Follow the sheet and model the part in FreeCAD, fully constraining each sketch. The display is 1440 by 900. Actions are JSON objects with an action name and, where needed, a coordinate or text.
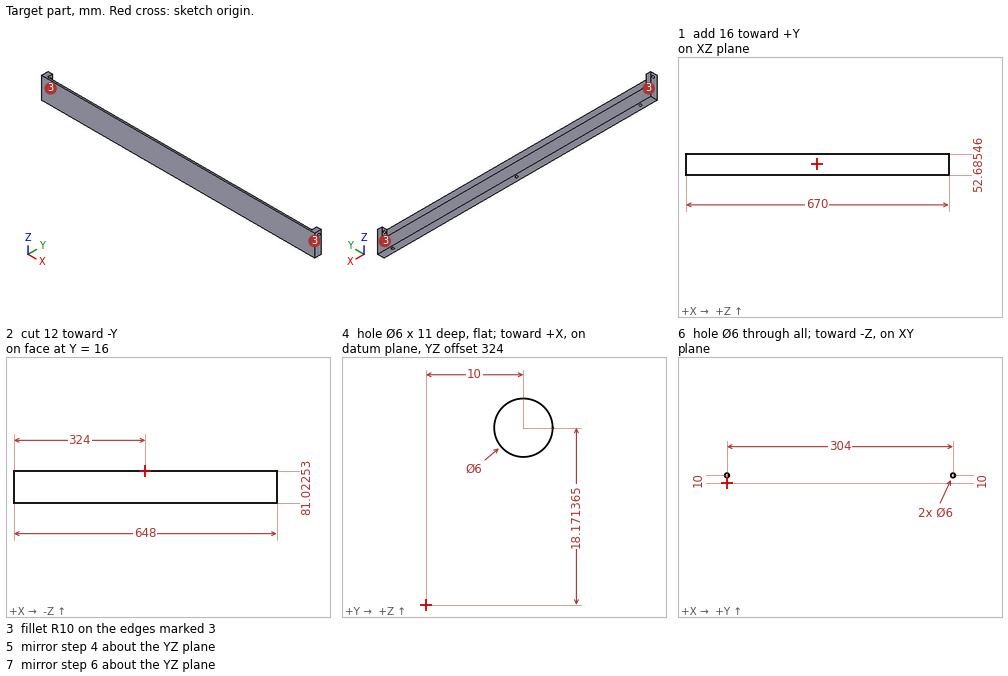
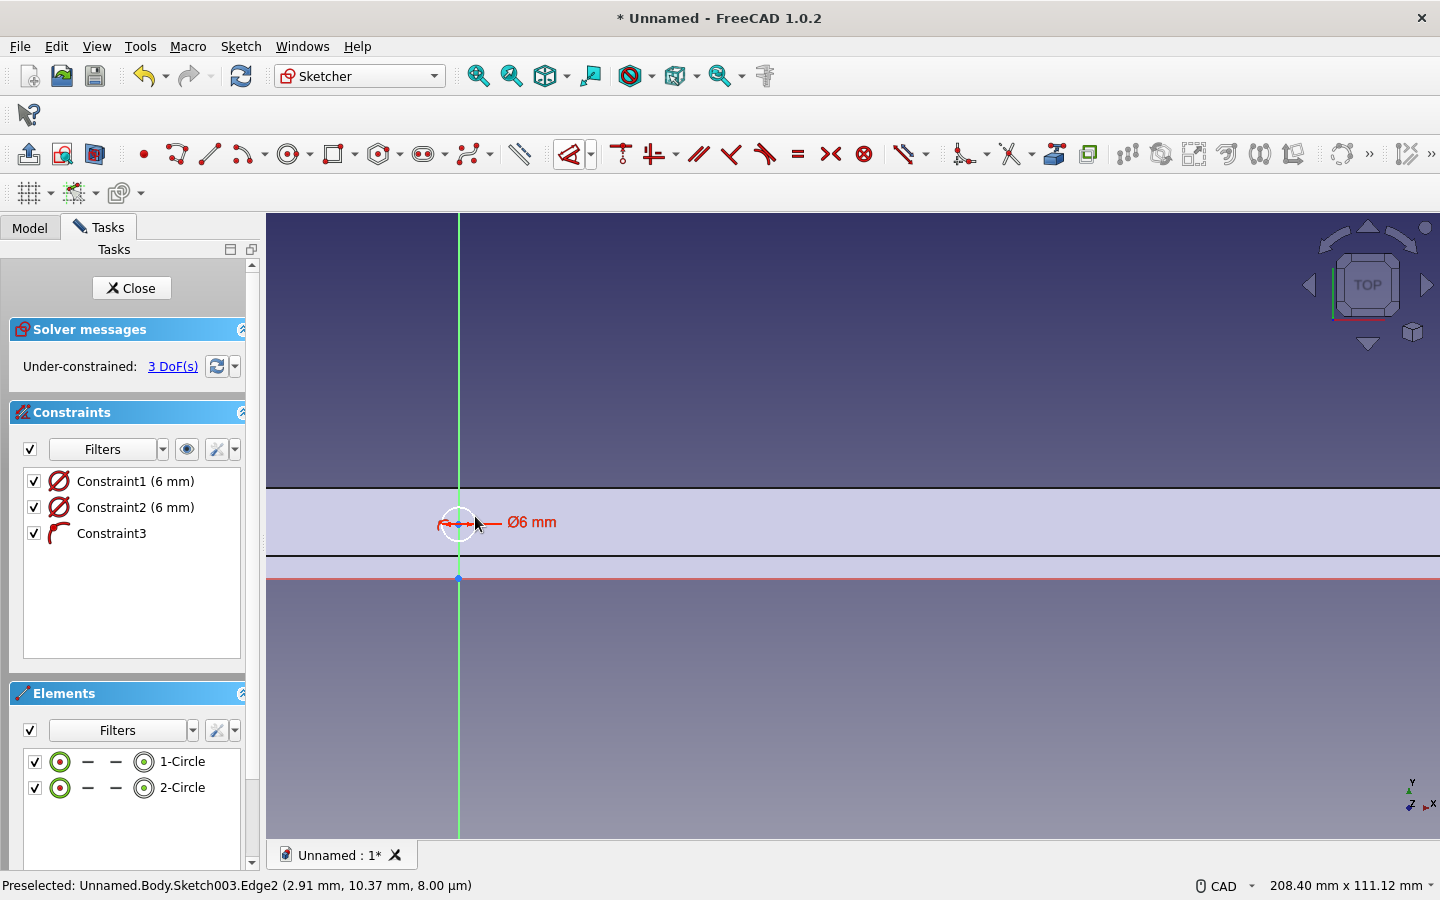
{"action": "scroll", "coordinate": [476, 517], "scroll_direction": "down", "scroll_amount": 5}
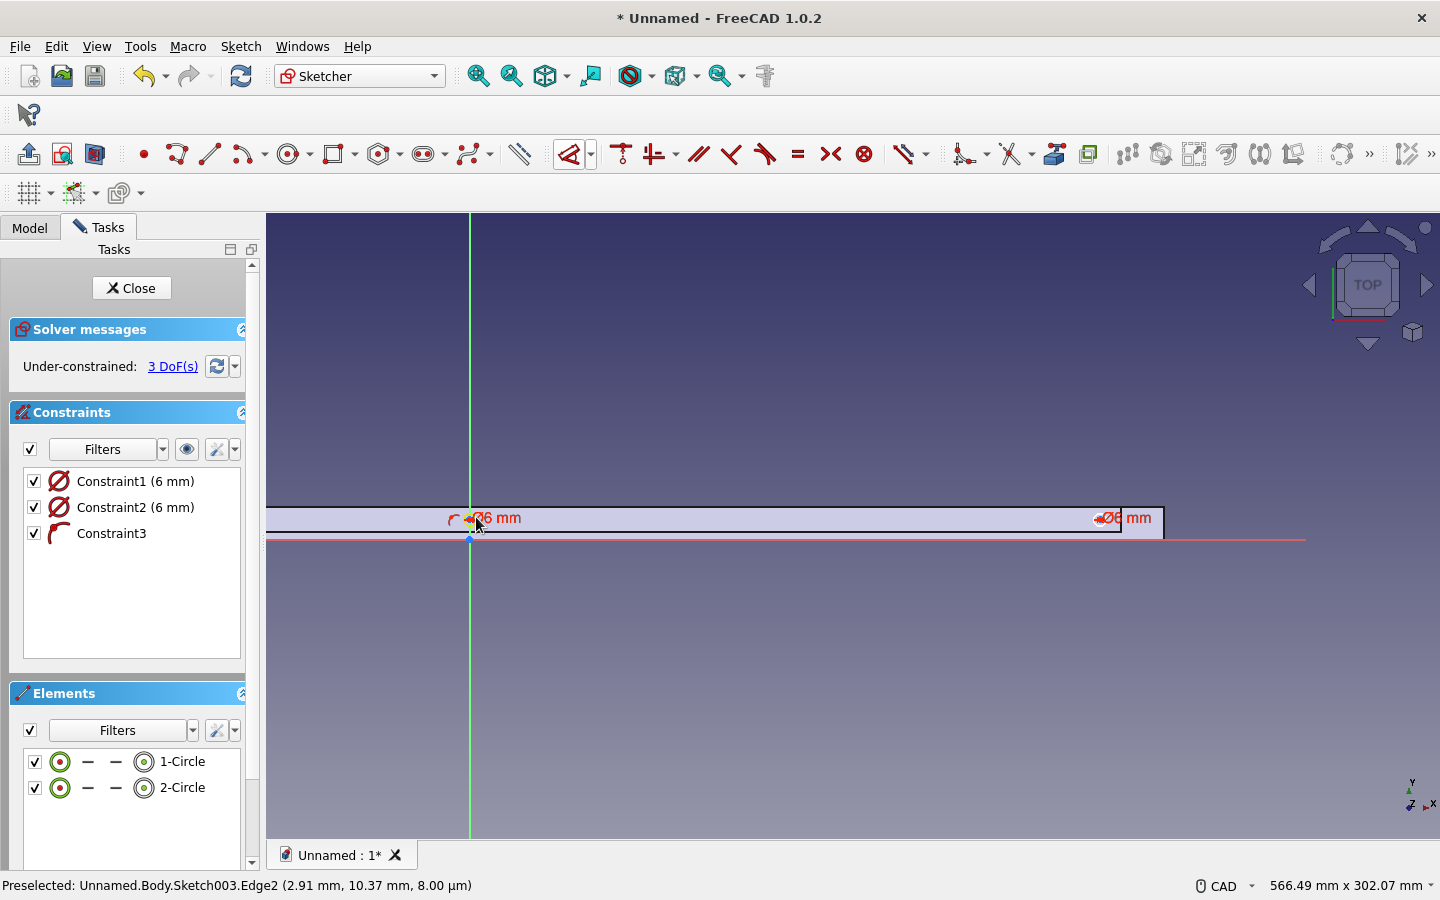
{"action": "scroll", "coordinate": [1100, 520], "scroll_direction": "up", "scroll_amount": 4}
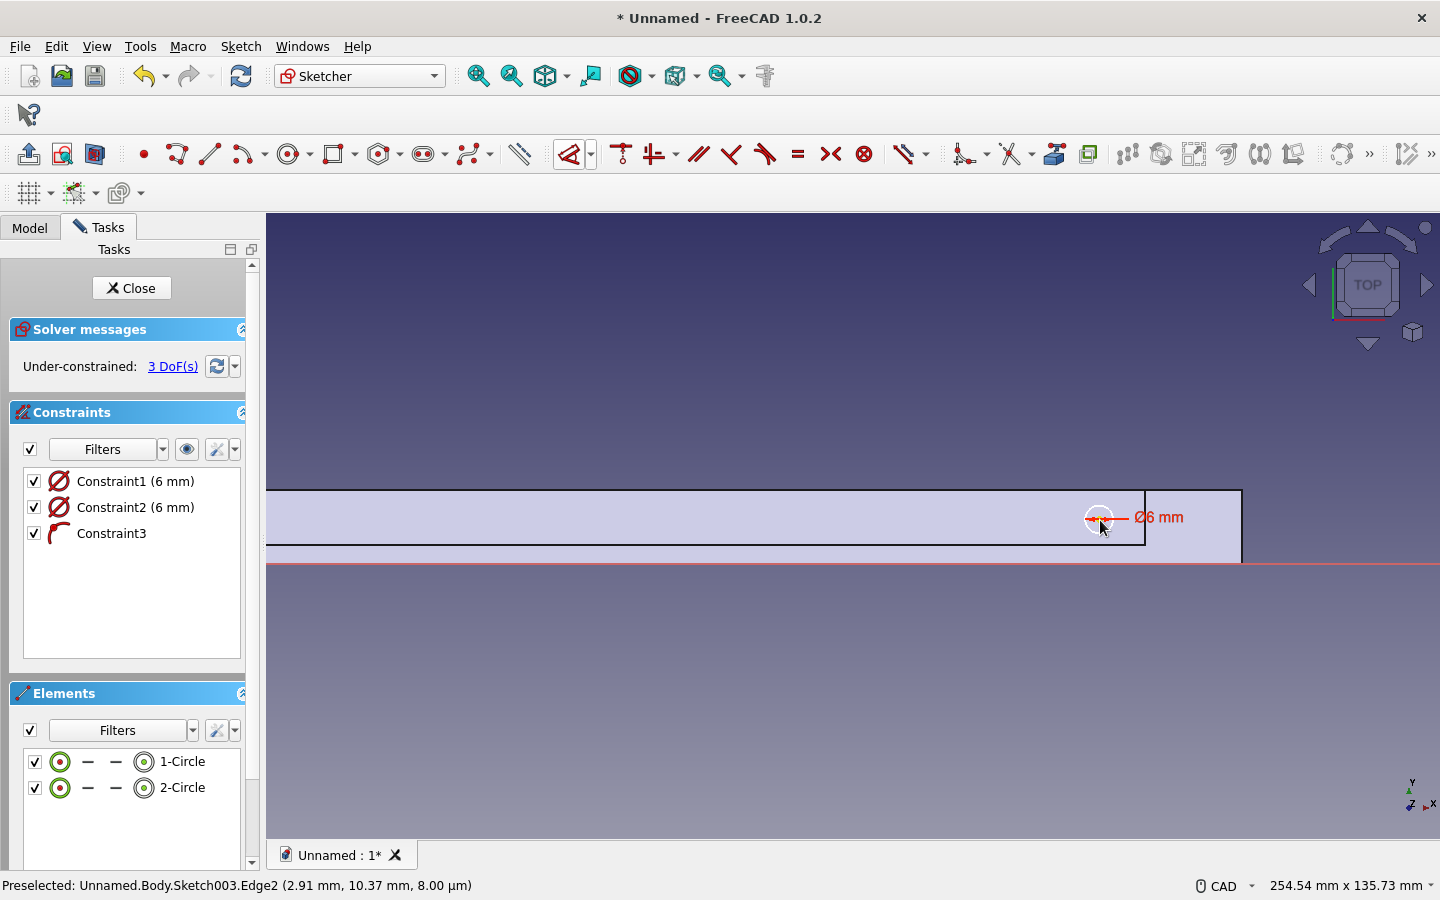
{"action": "left_click", "coordinate": [1099, 519]}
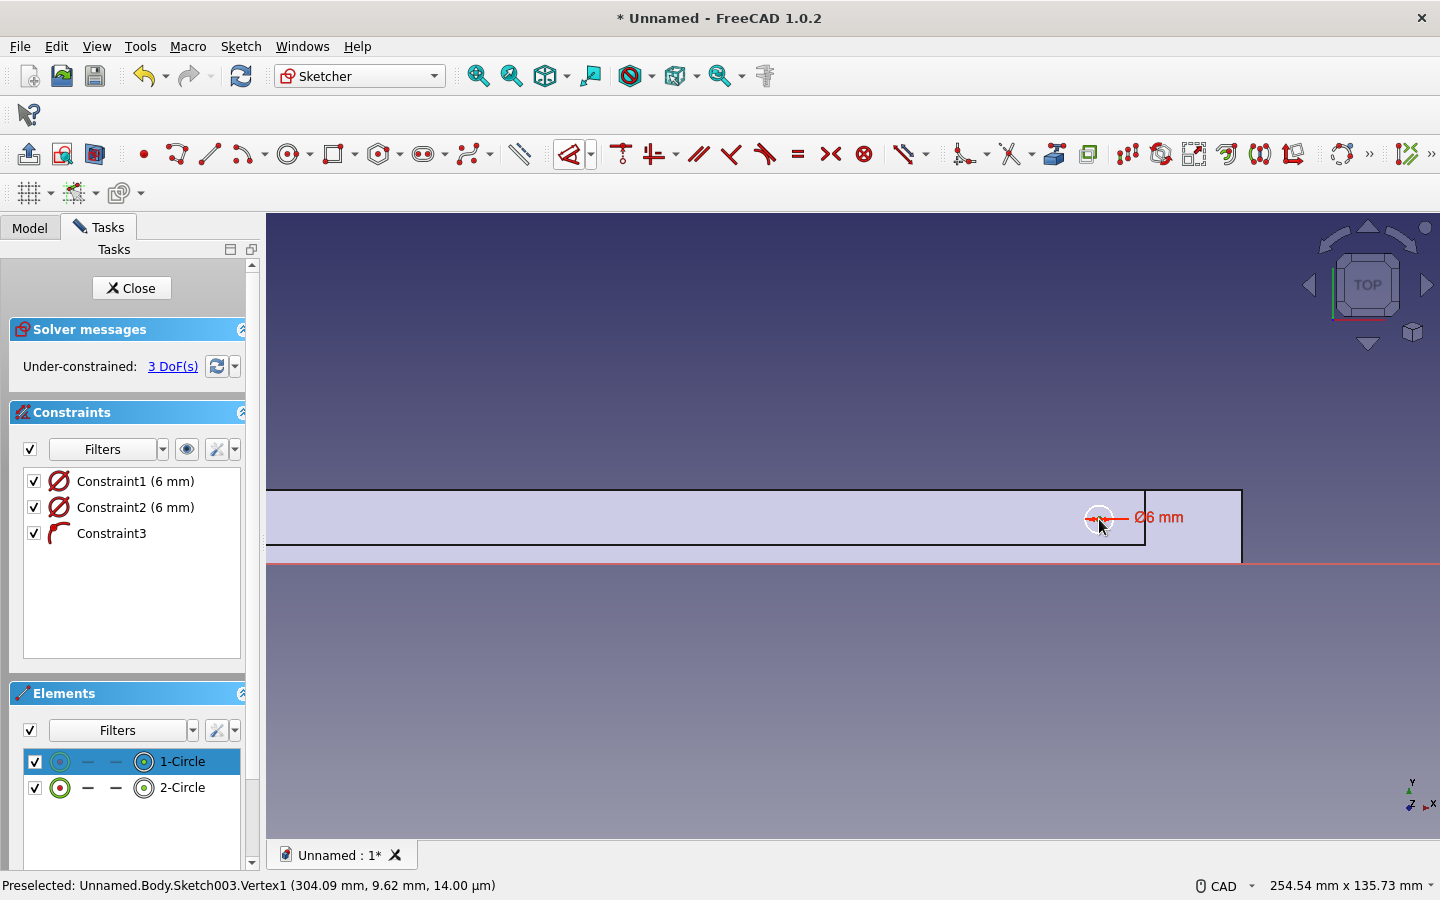
{"action": "left_click", "coordinate": [590, 154]}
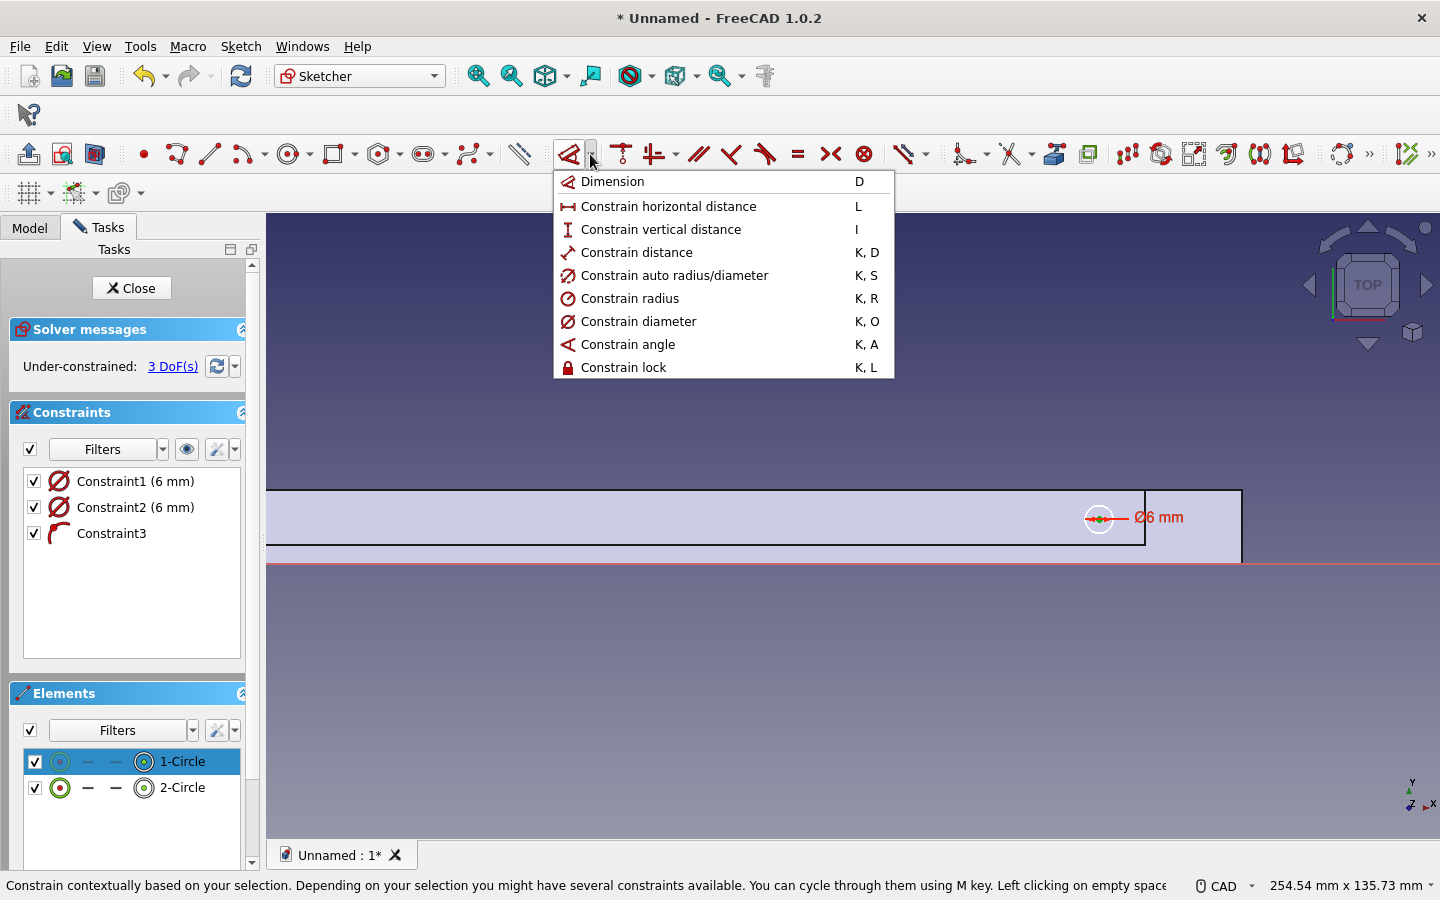
{"action": "left_click", "coordinate": [724, 230]}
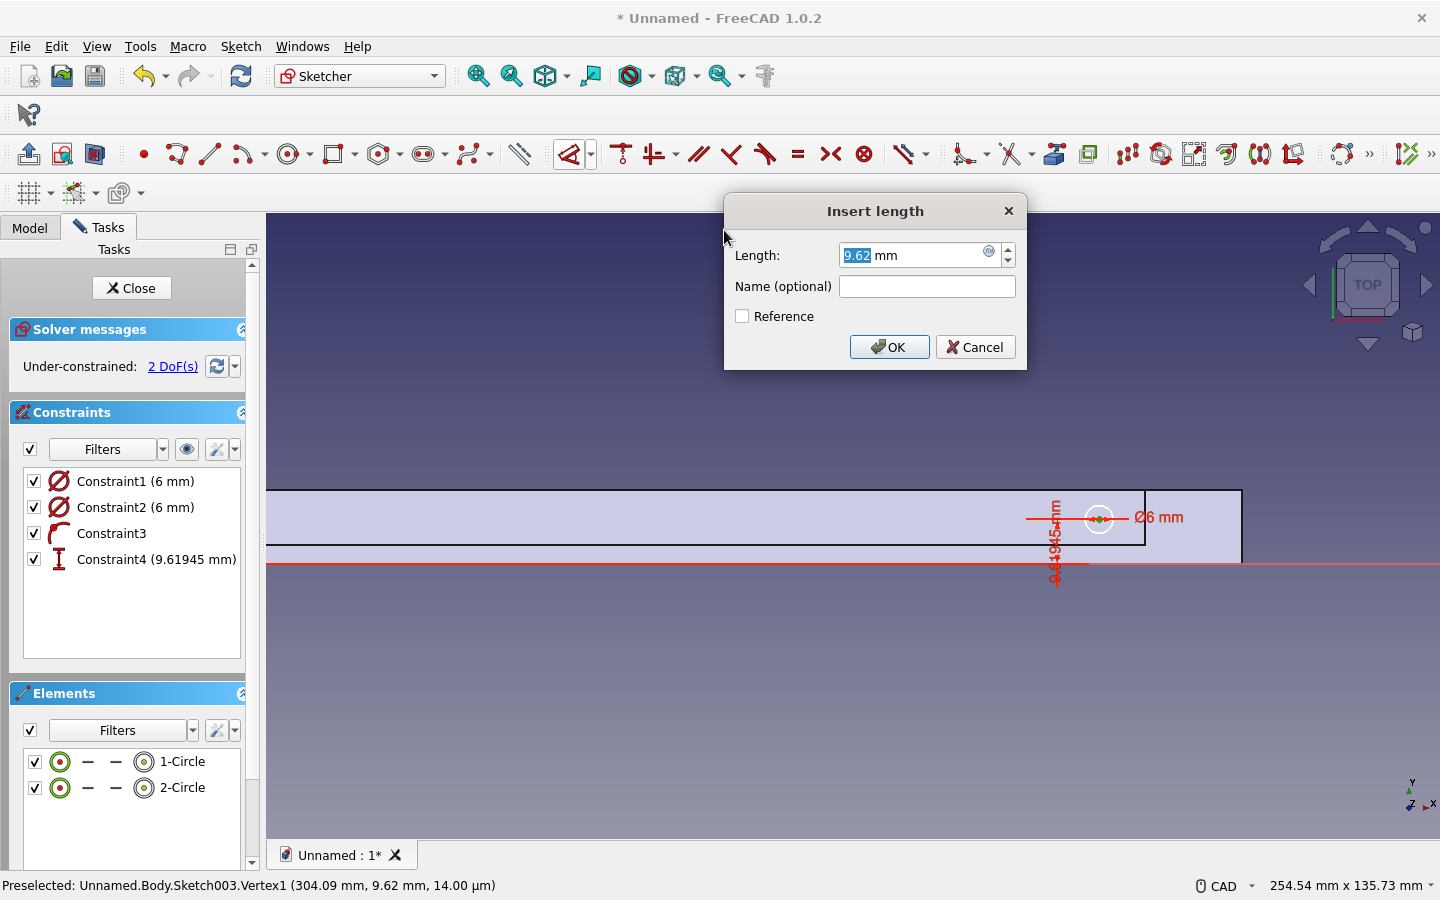
{"action": "type", "text": "10"}
{"action": "key", "text": "Return"}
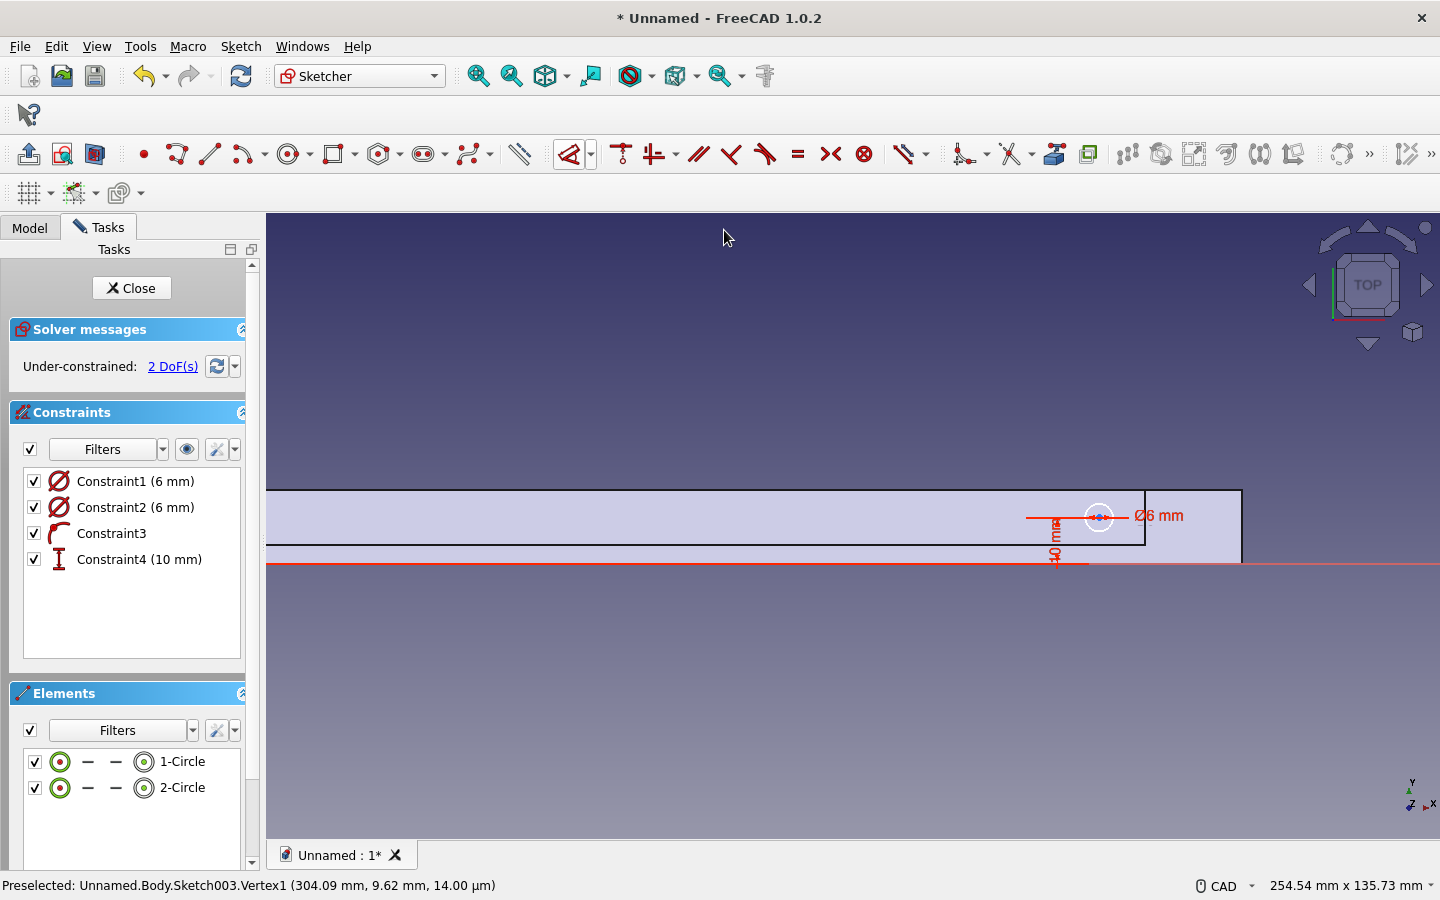
{"action": "scroll", "coordinate": [1100, 520], "scroll_direction": "down", "scroll_amount": 4}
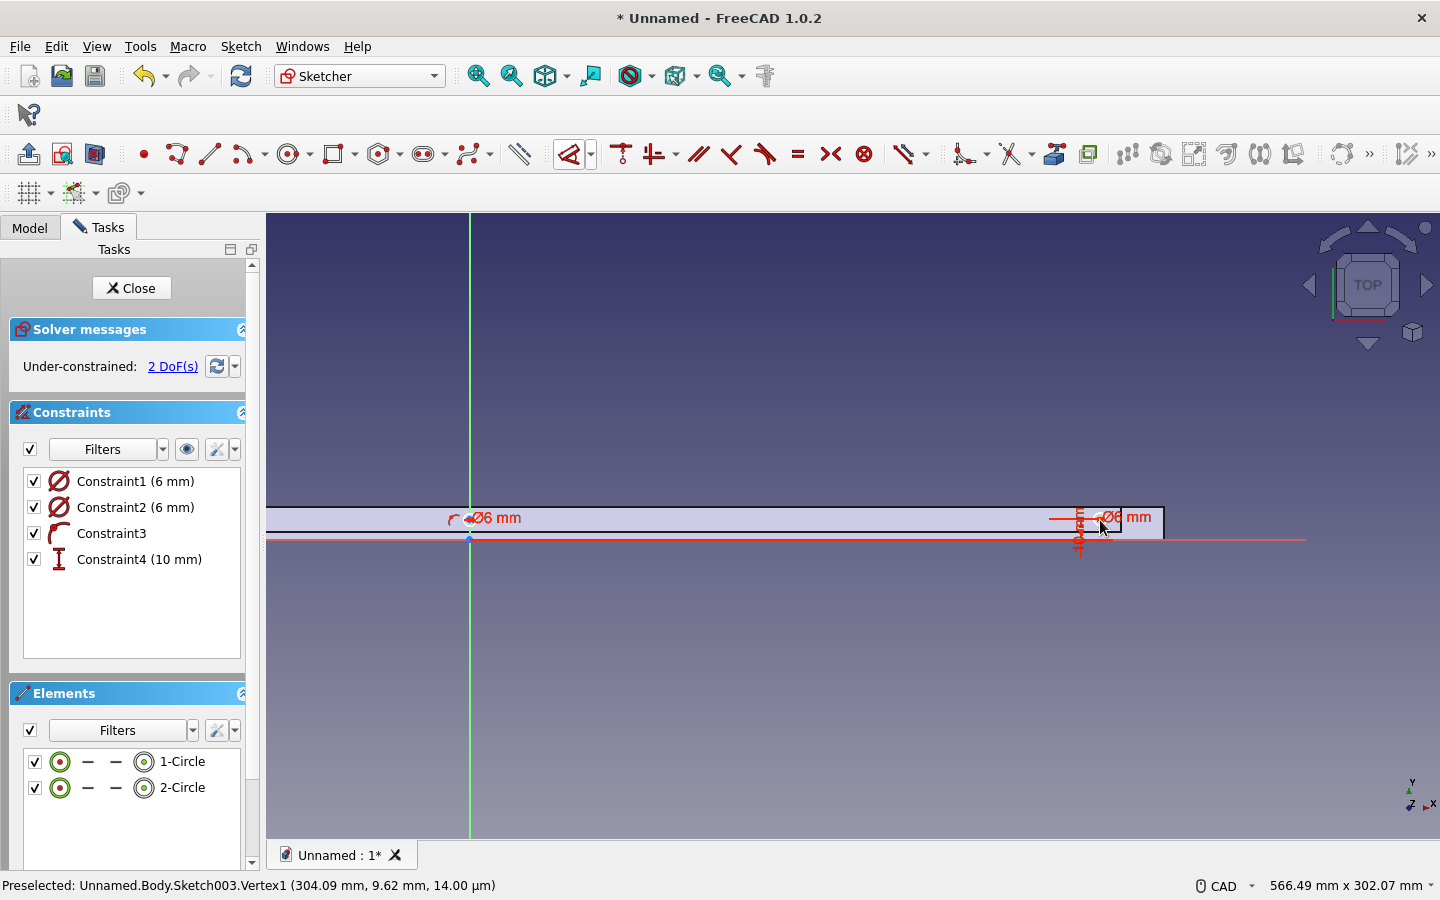
{"action": "scroll", "coordinate": [470, 520], "scroll_direction": "up", "scroll_amount": 4}